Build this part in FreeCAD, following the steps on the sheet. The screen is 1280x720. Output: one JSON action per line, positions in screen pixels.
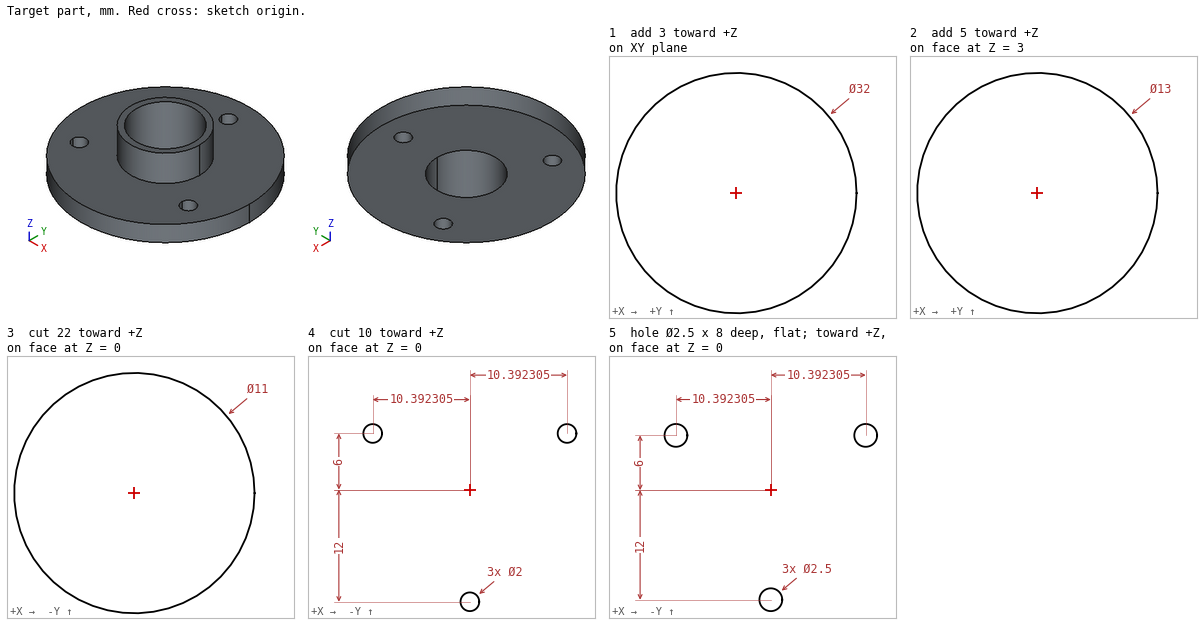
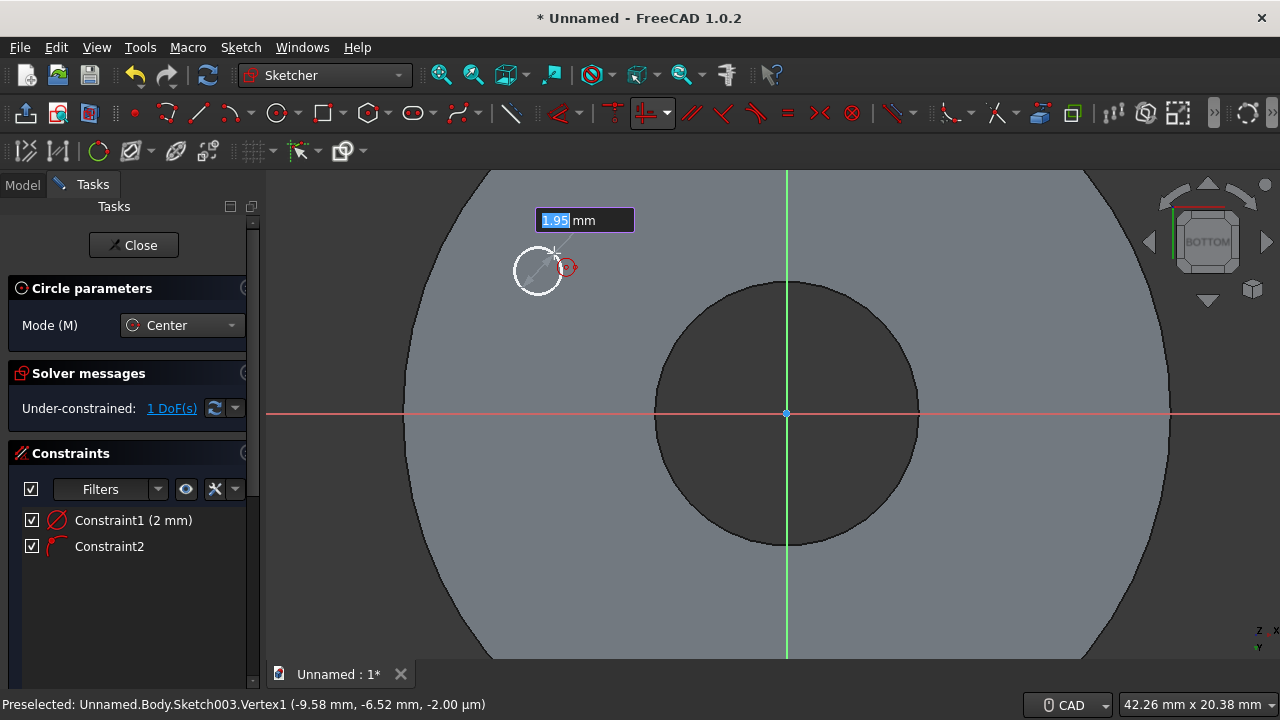
{"action": "type", "text": "2"}
{"action": "key", "text": "Return"}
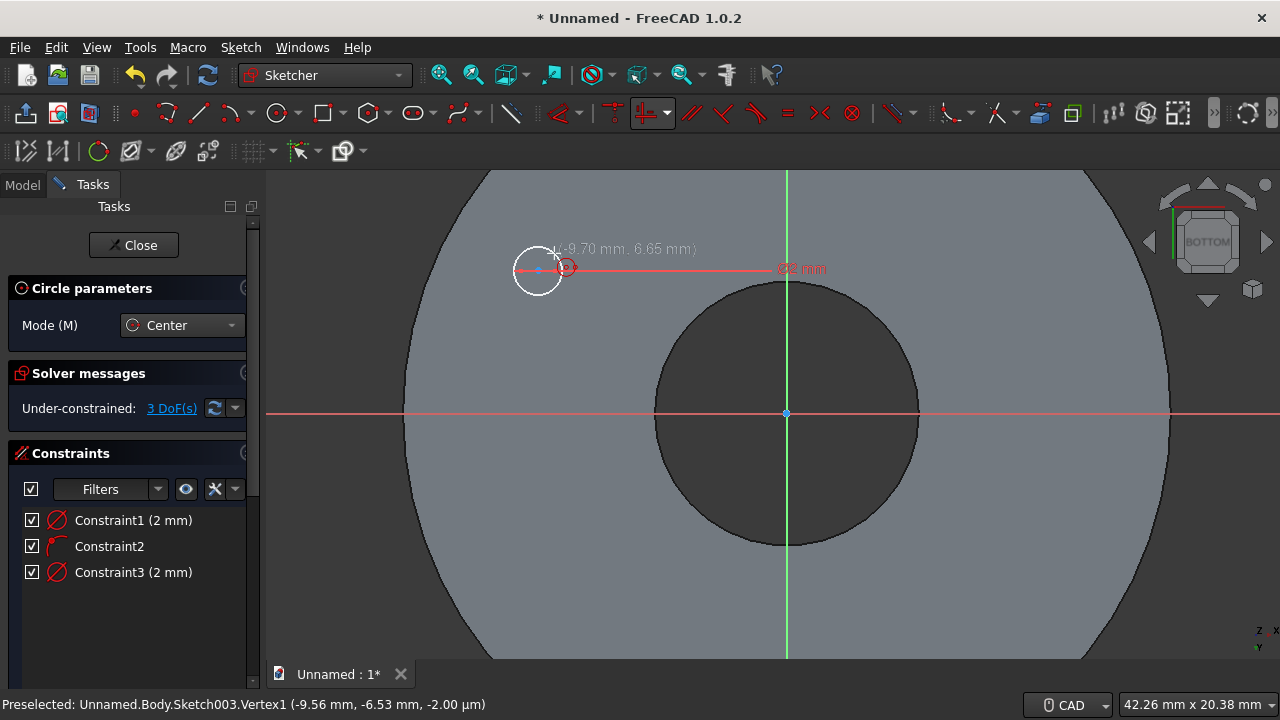
{"action": "left_click", "coordinate": [1036, 270]}
{"action": "mouse_move", "coordinate": [1053, 253]}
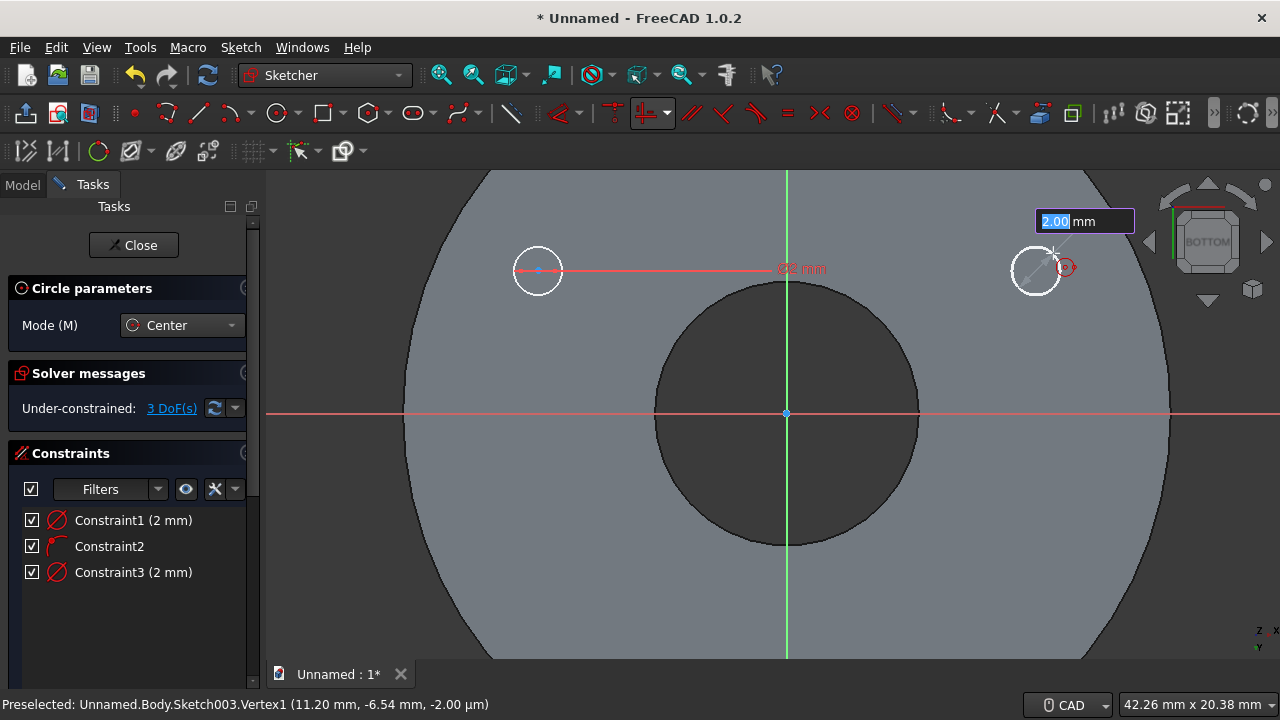
{"action": "type", "text": "2"}
{"action": "key", "text": "Return"}
{"action": "key", "text": "Escape"}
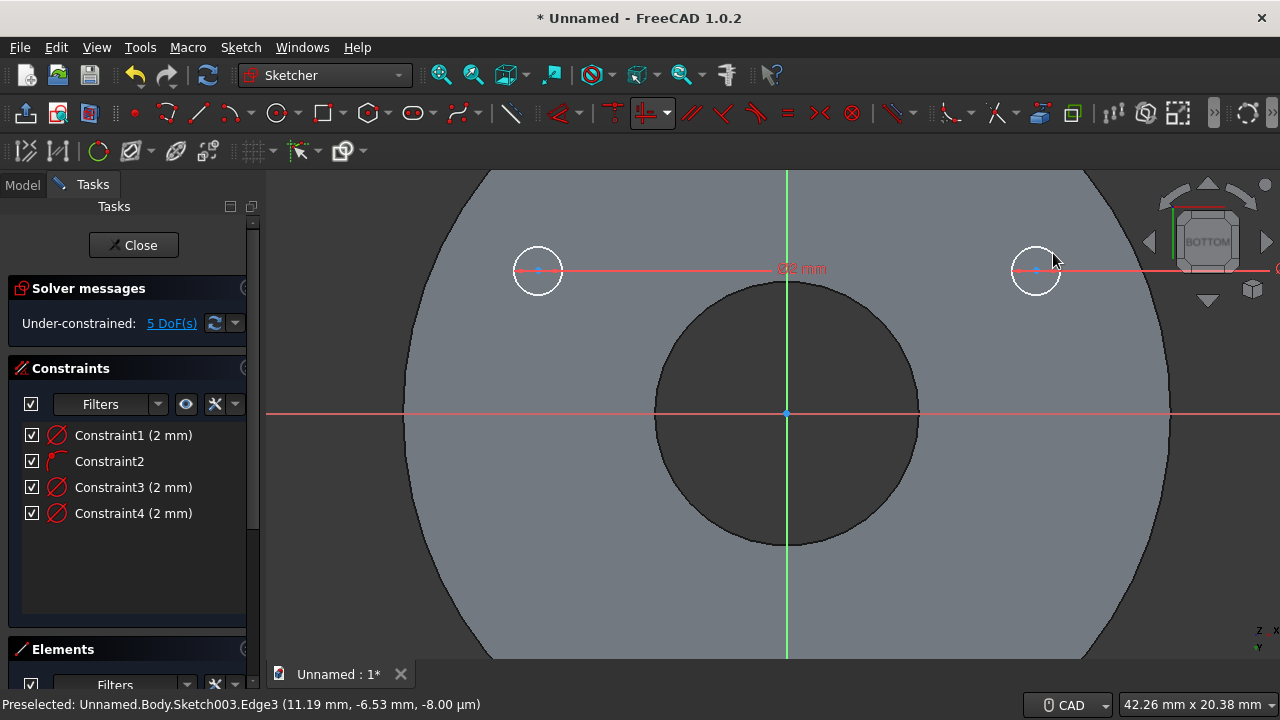
{"action": "left_click", "coordinate": [538, 271]}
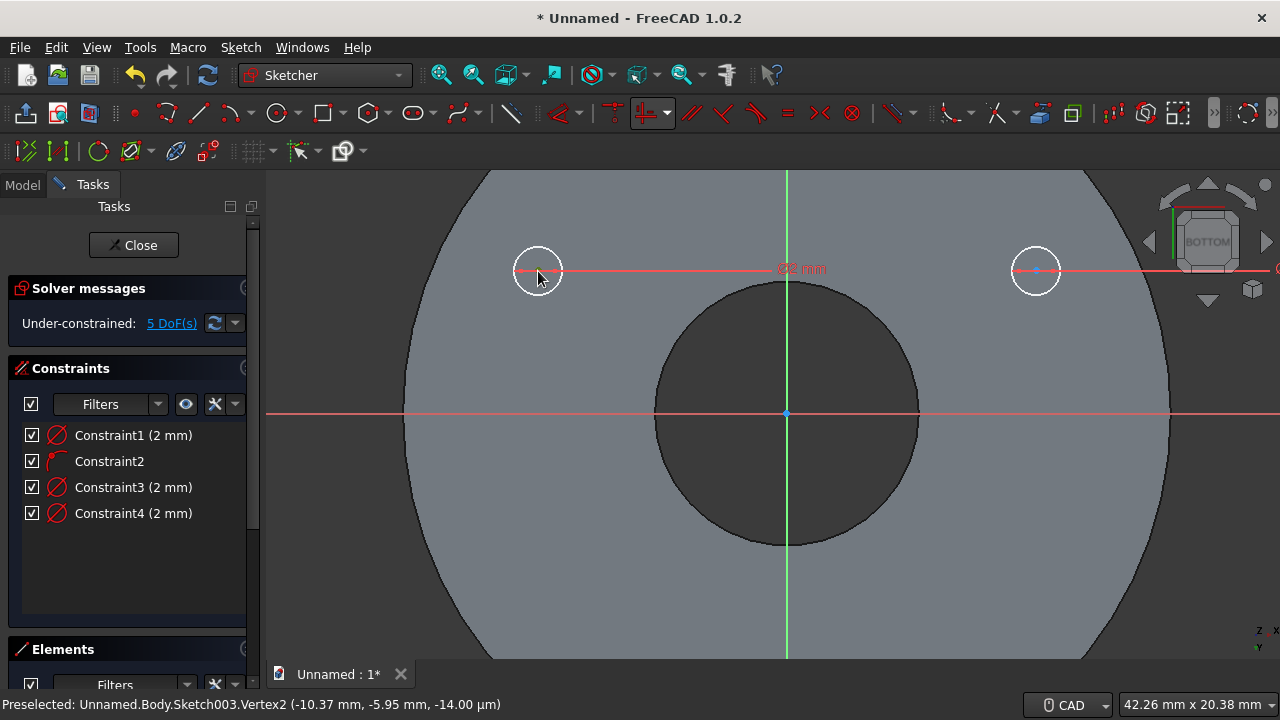
{"action": "left_click", "coordinate": [1036, 271]}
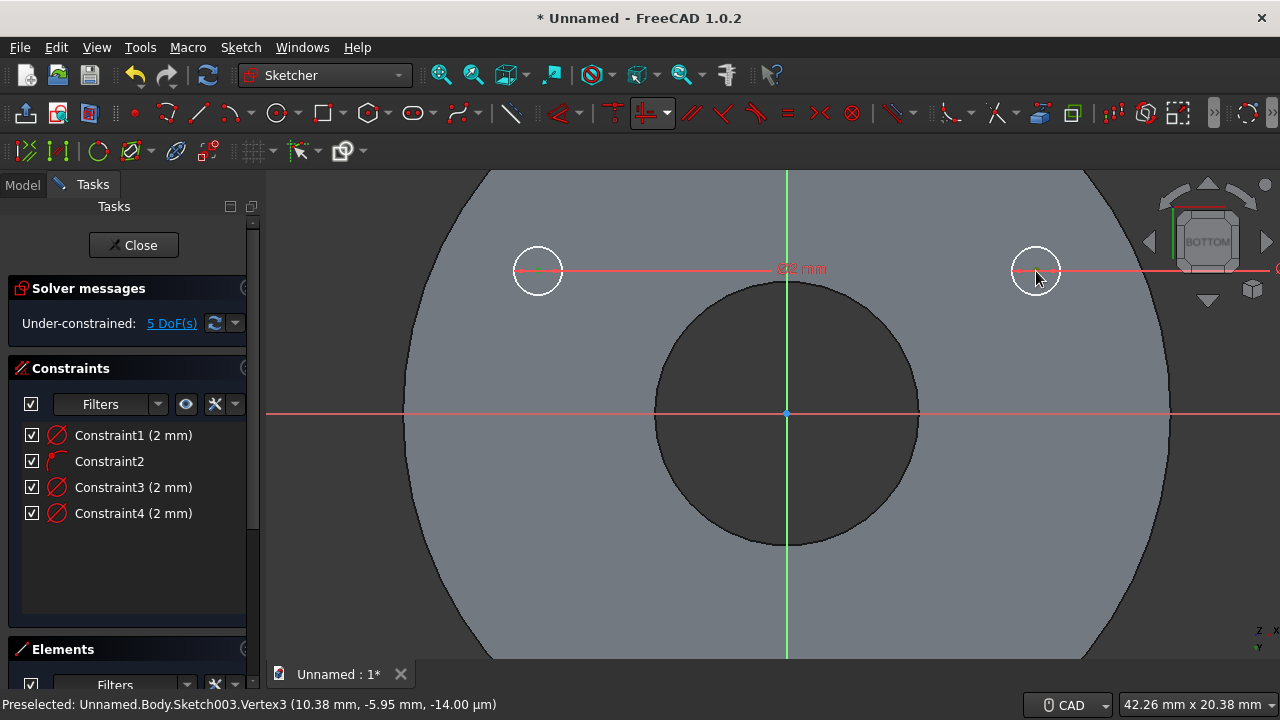
{"action": "left_click", "coordinate": [670, 114]}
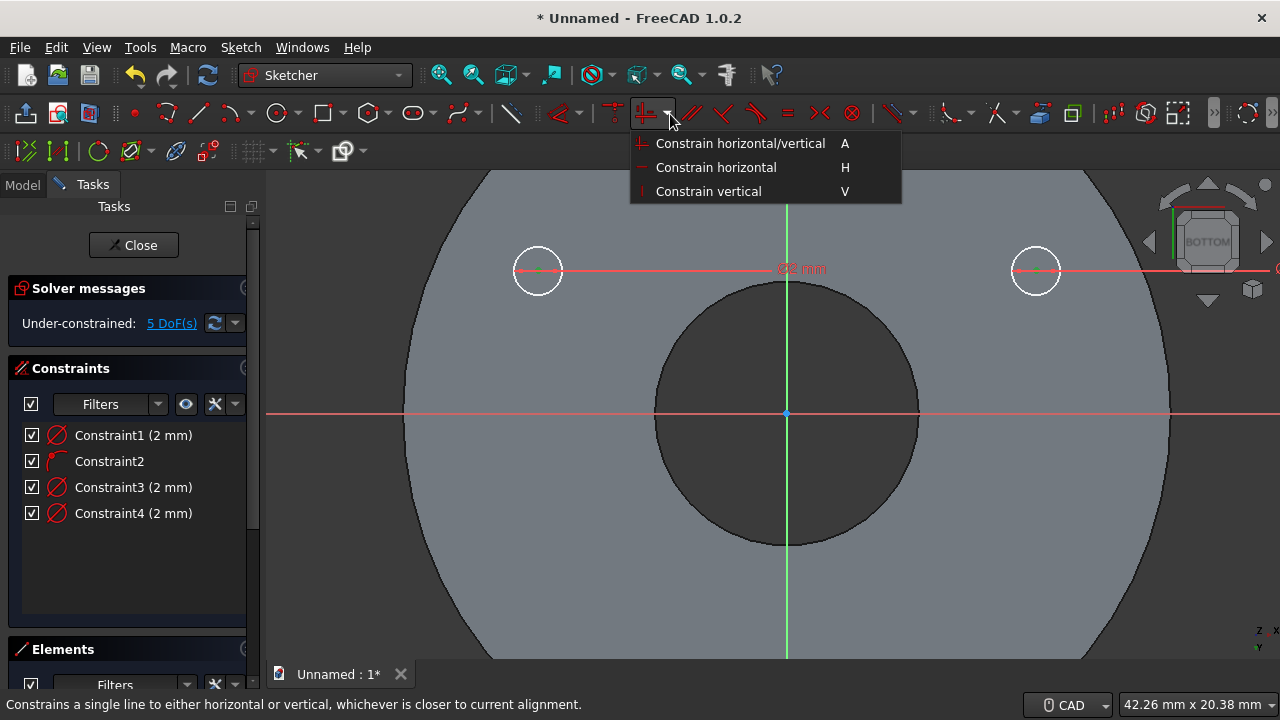
{"action": "left_click", "coordinate": [766, 167]}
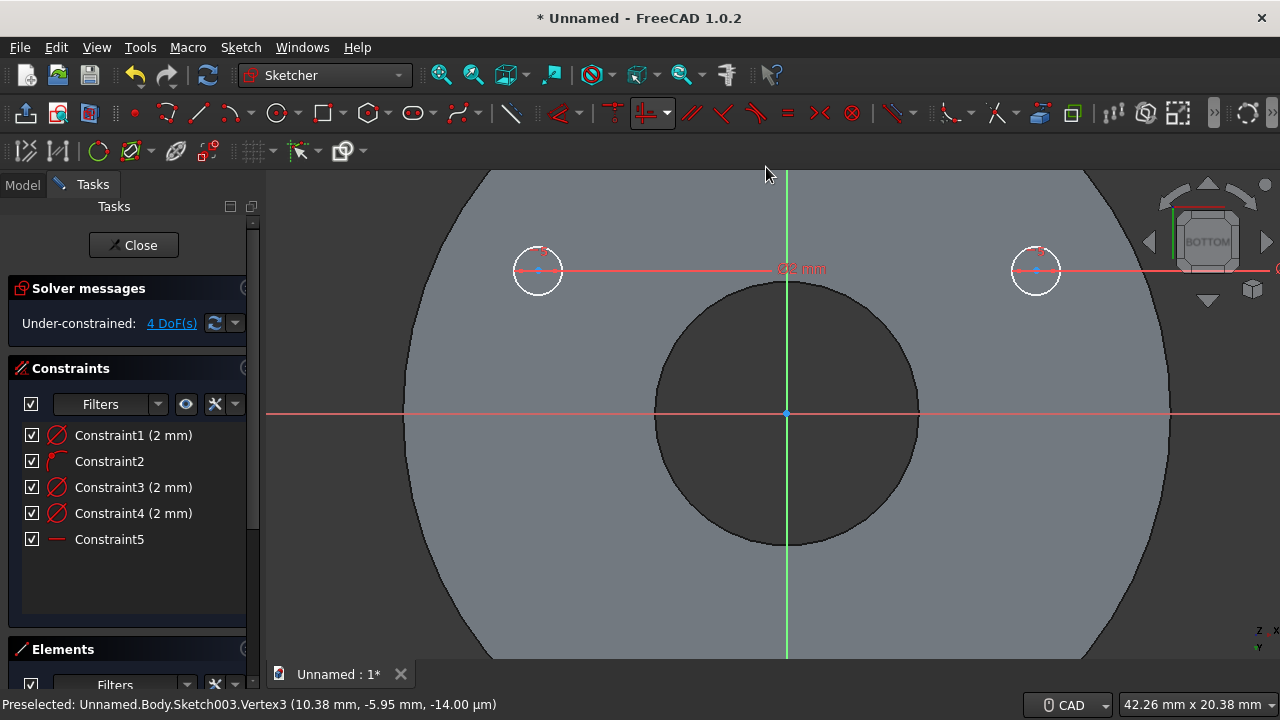
{"action": "left_click", "coordinate": [558, 114]}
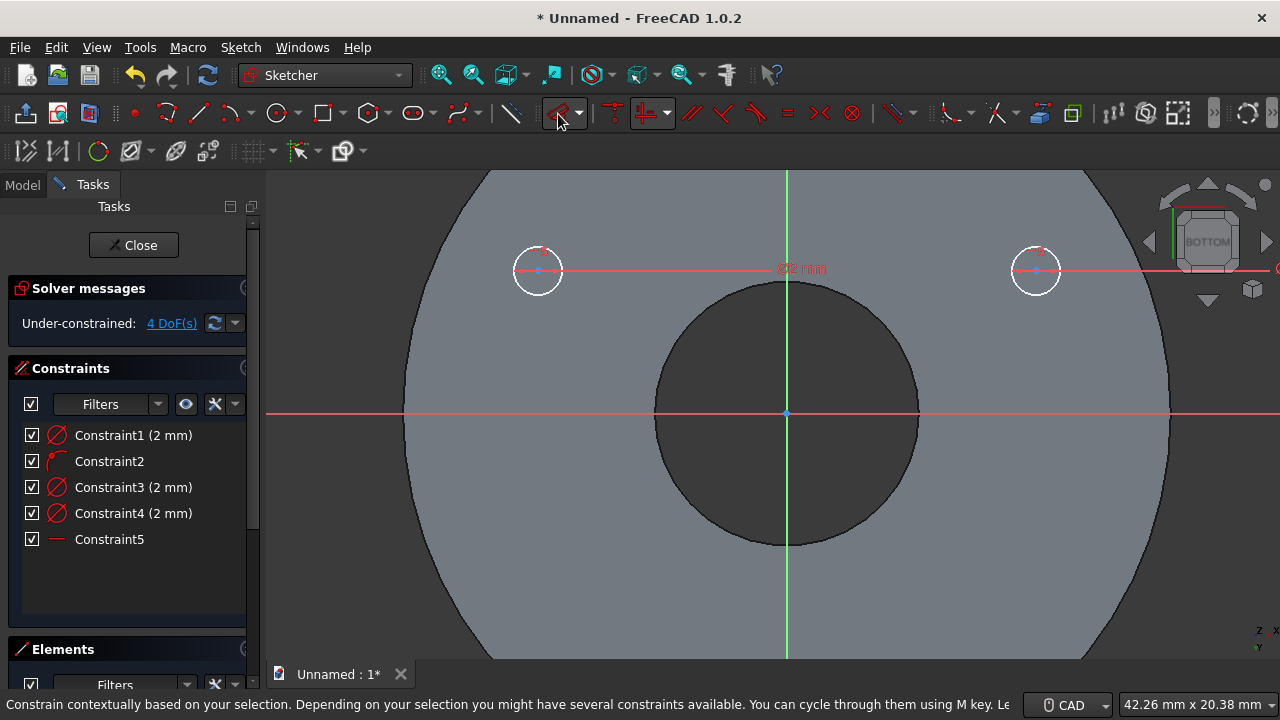
{"action": "left_click", "coordinate": [538, 271]}
{"action": "left_click", "coordinate": [504, 342]}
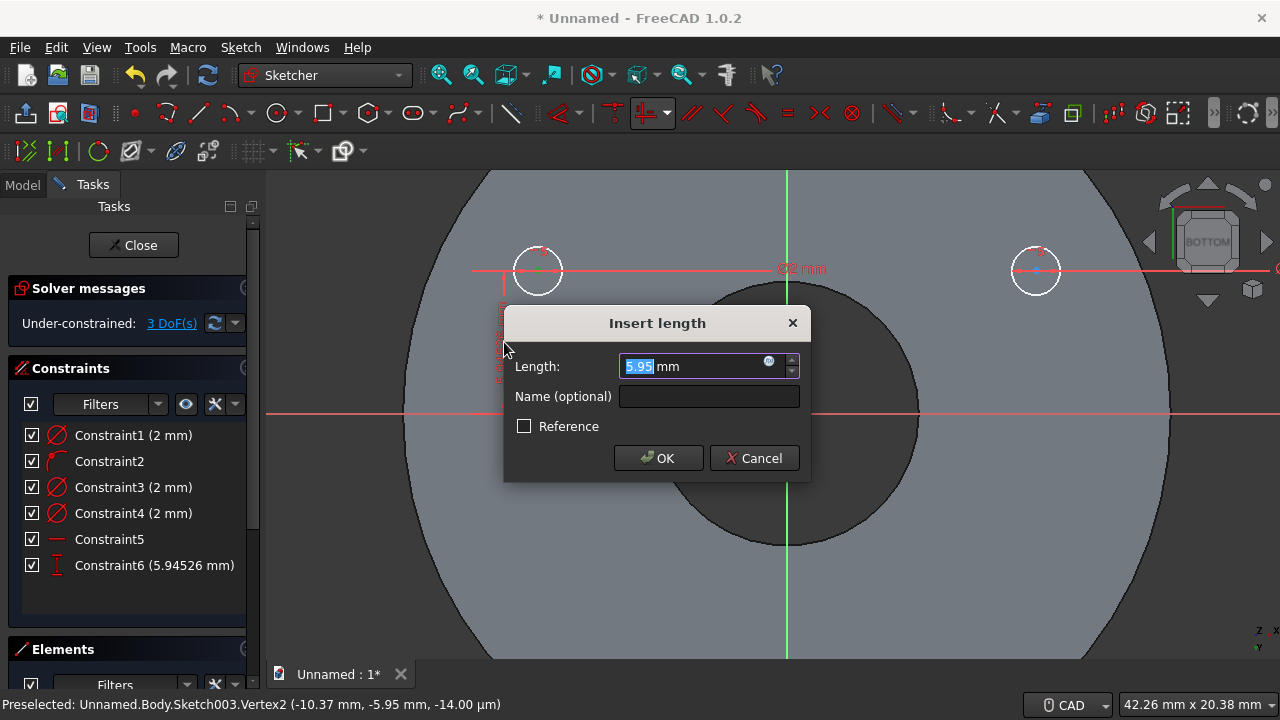
{"action": "type", "text": "6"}
{"action": "key", "text": "Return"}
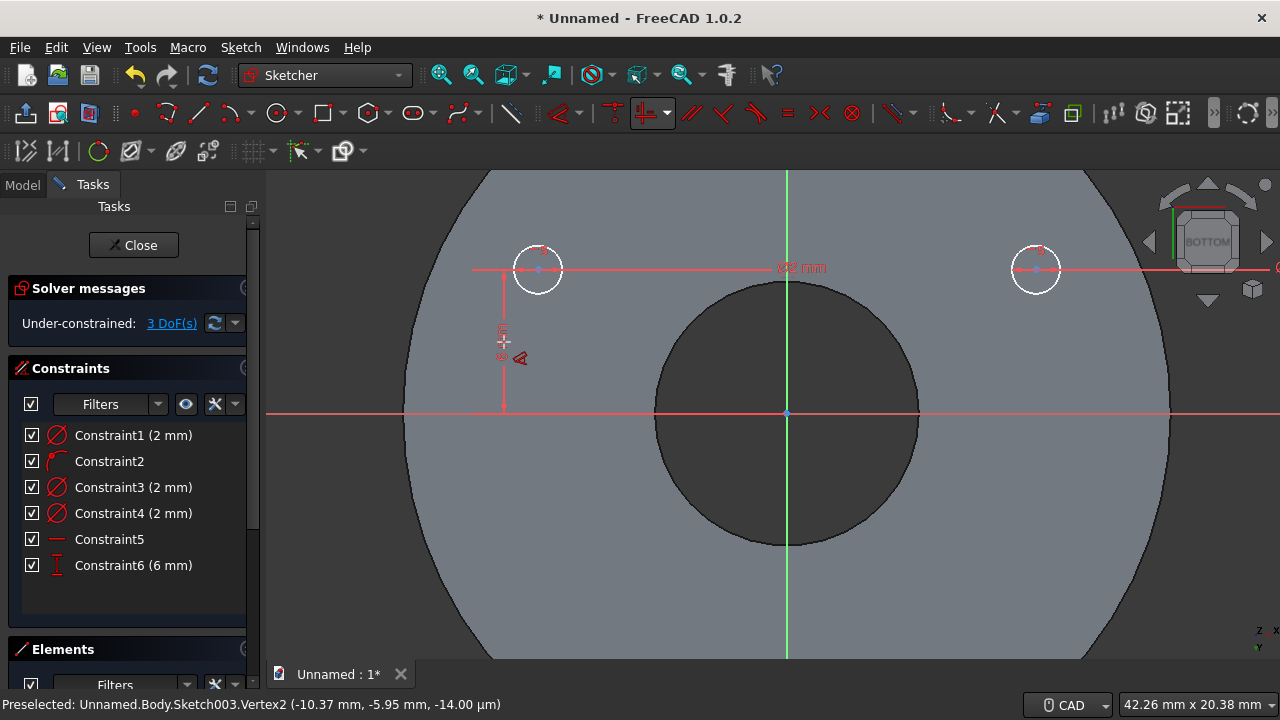
{"action": "scroll", "coordinate": [537, 270], "scroll_direction": "down", "scroll_amount": 2}